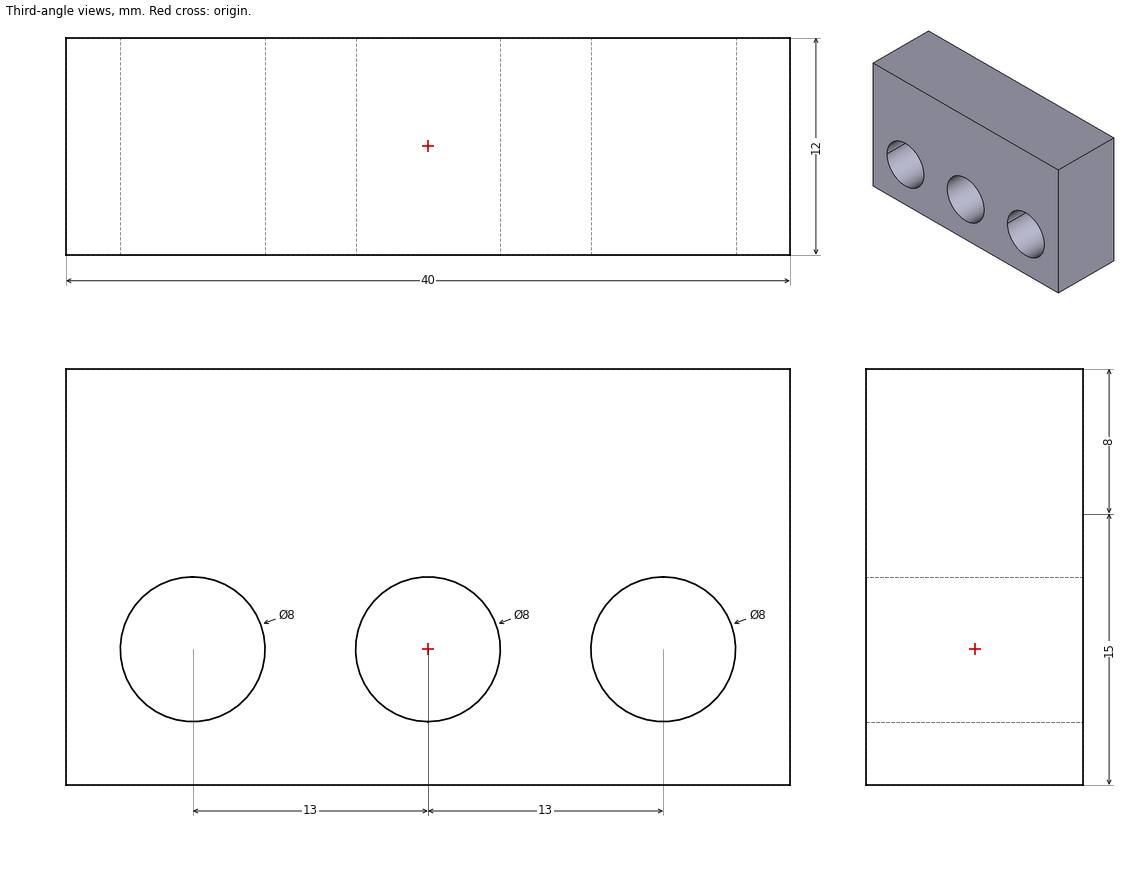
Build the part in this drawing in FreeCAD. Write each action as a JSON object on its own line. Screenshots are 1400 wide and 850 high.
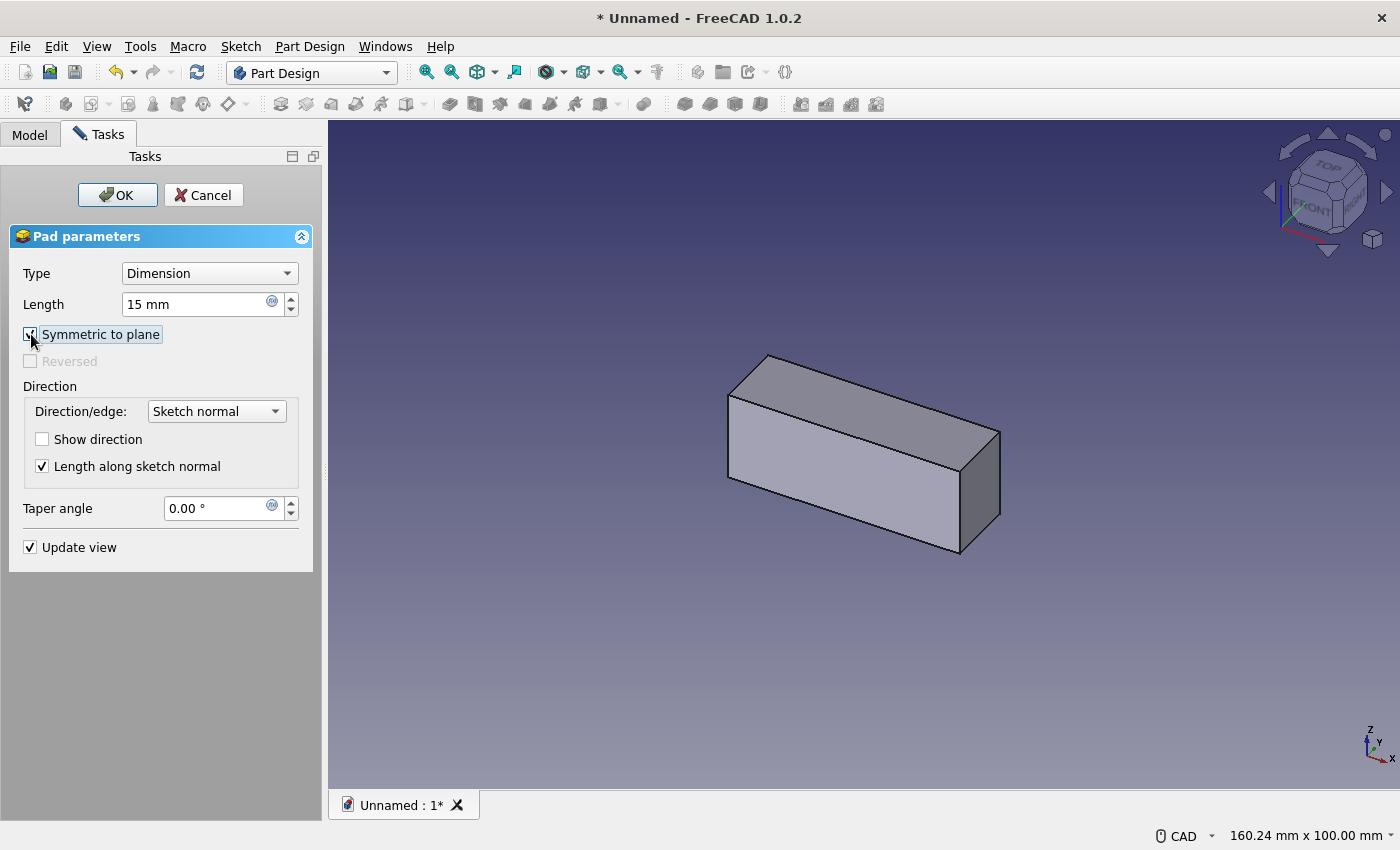
{"action": "left_click", "coordinate": [118, 195]}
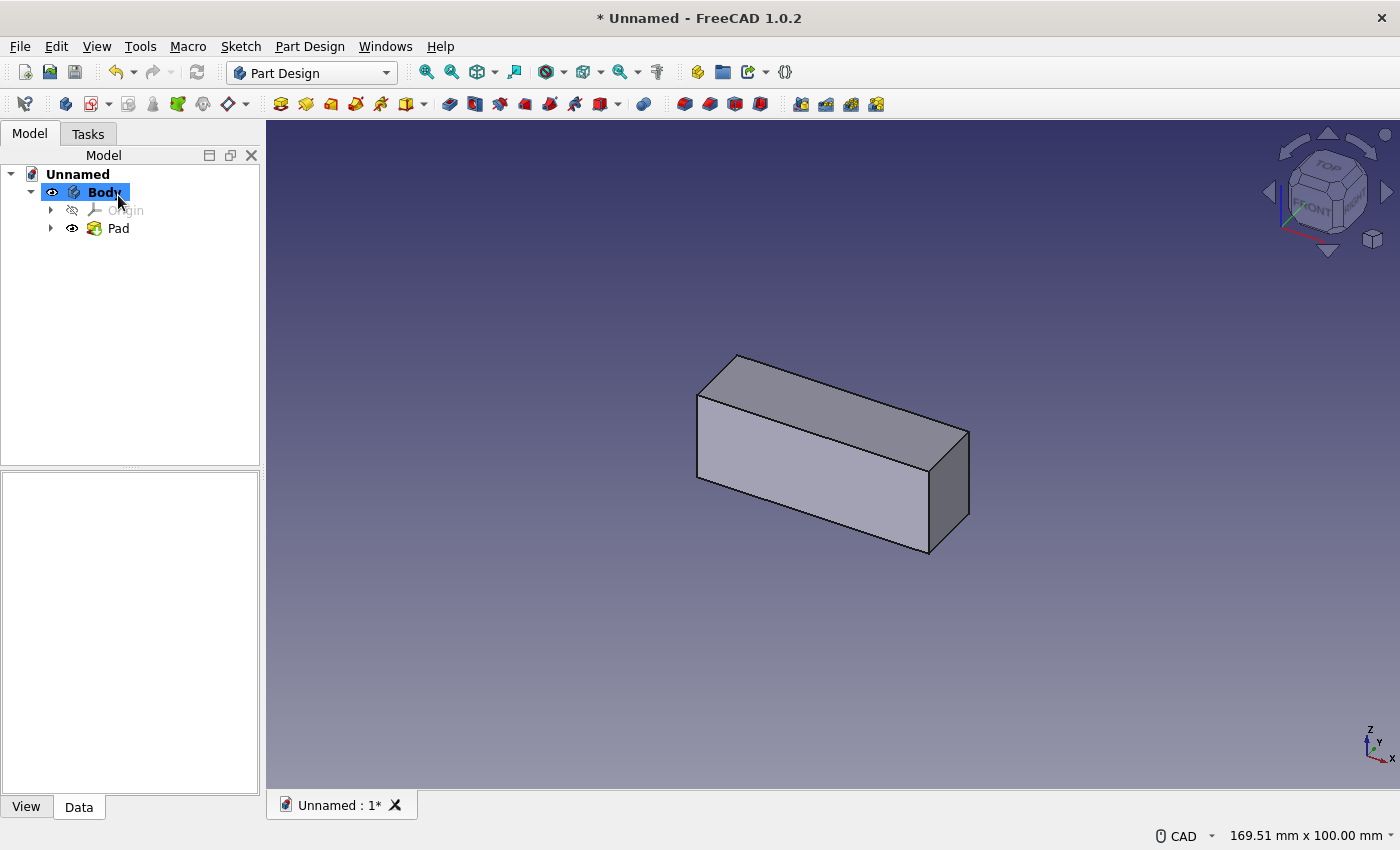
{"action": "key", "text": "v f"}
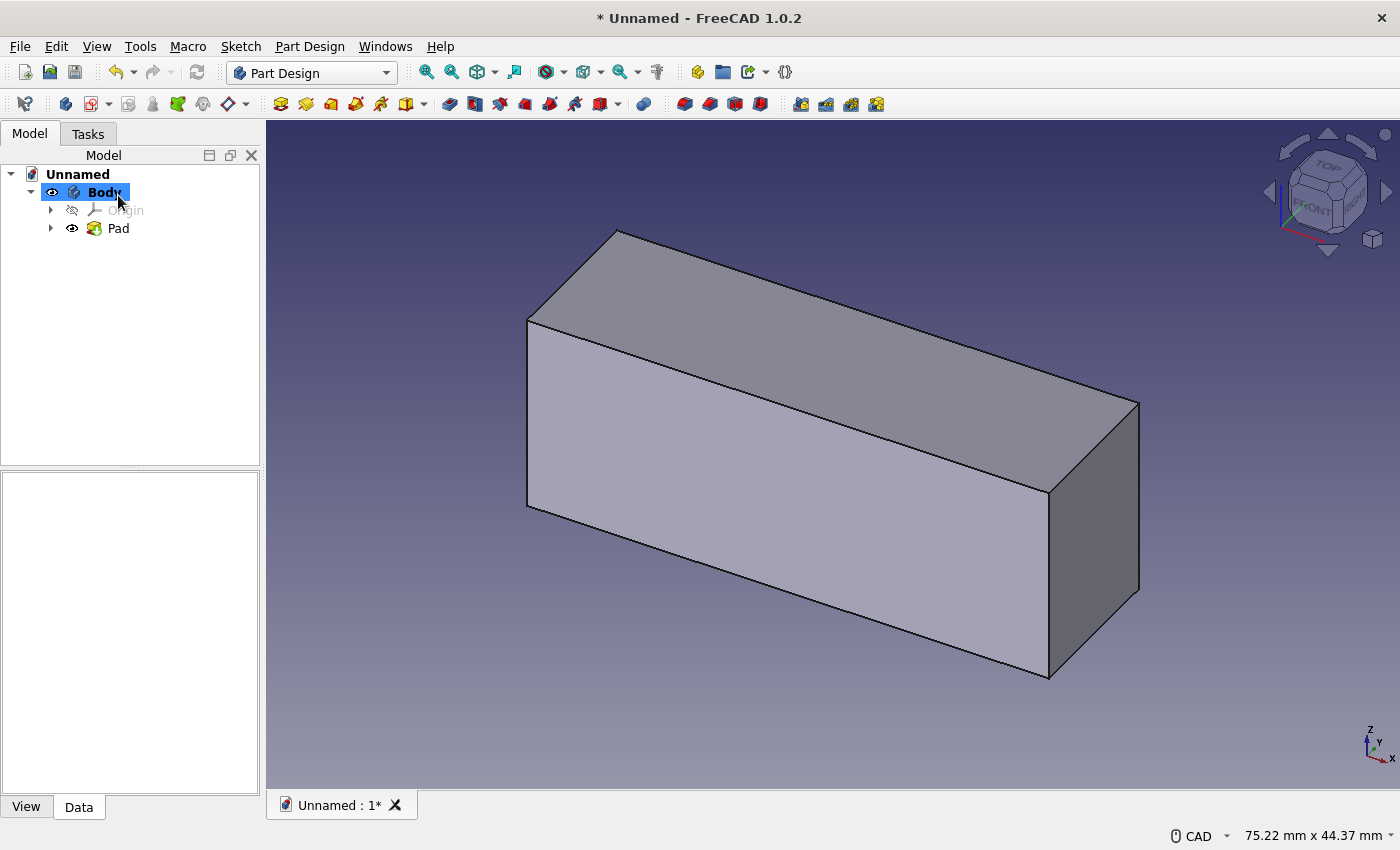
{"action": "key", "text": "4"}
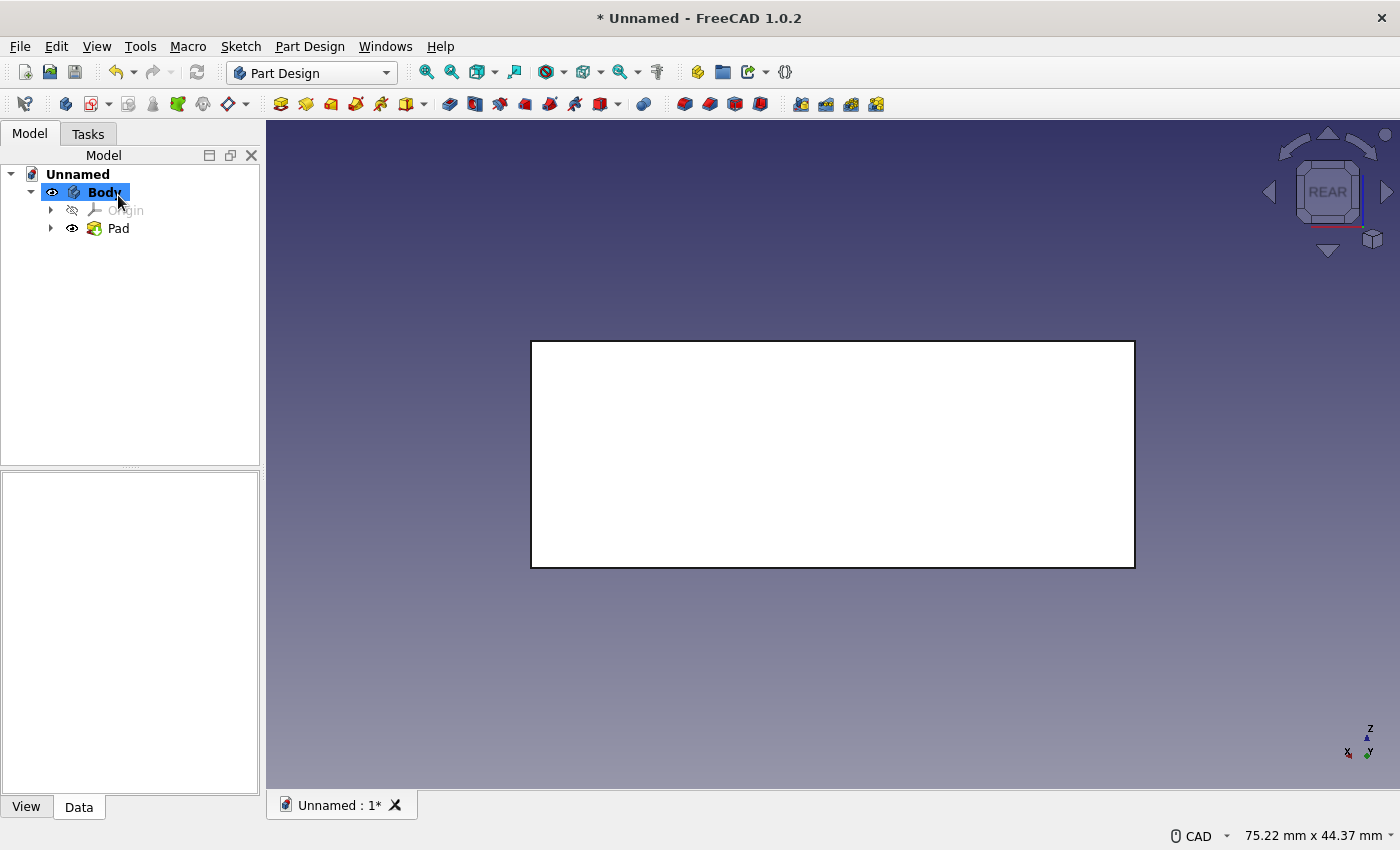
{"action": "left_click", "coordinate": [661, 453]}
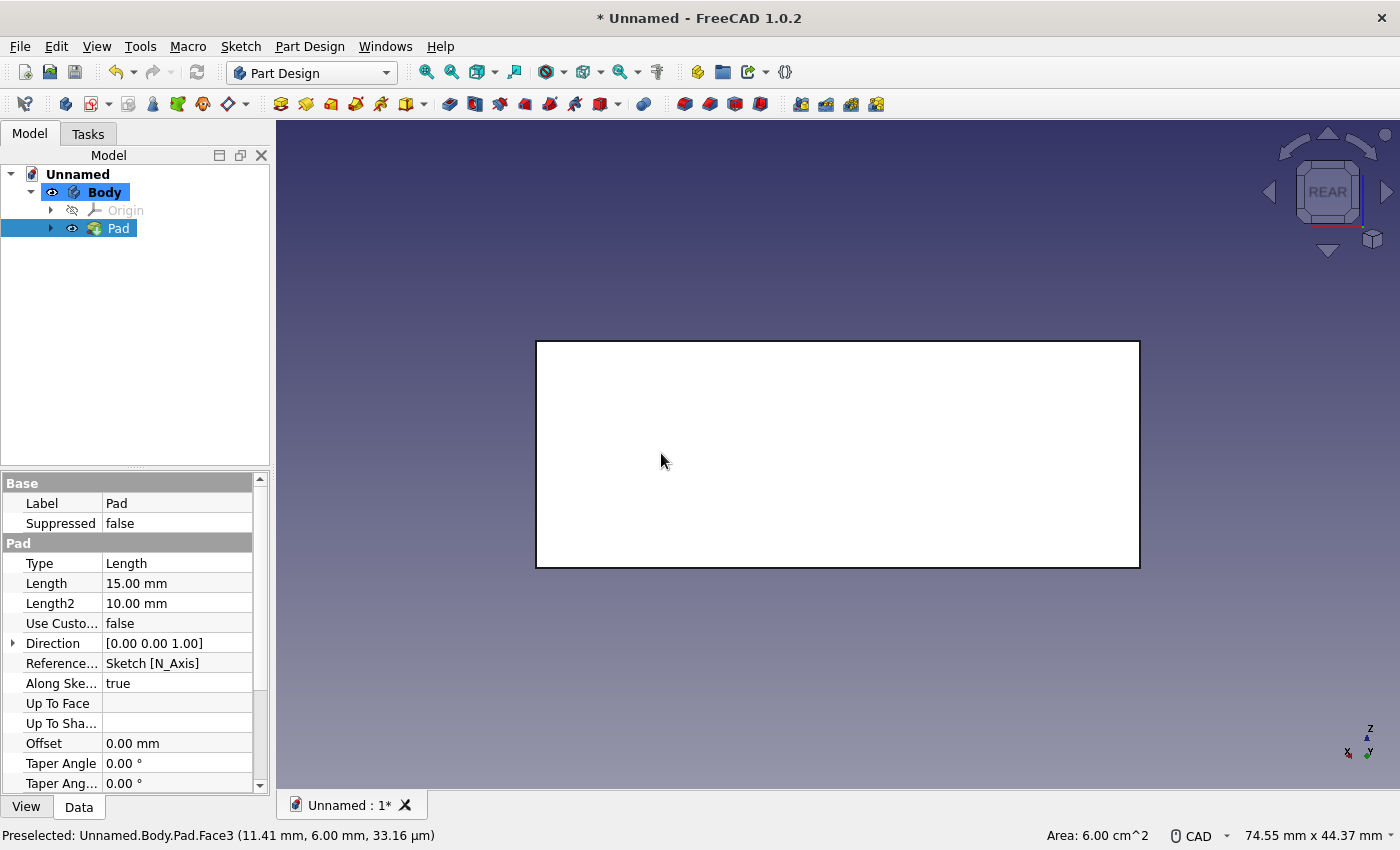
{"action": "left_click", "coordinate": [90, 104]}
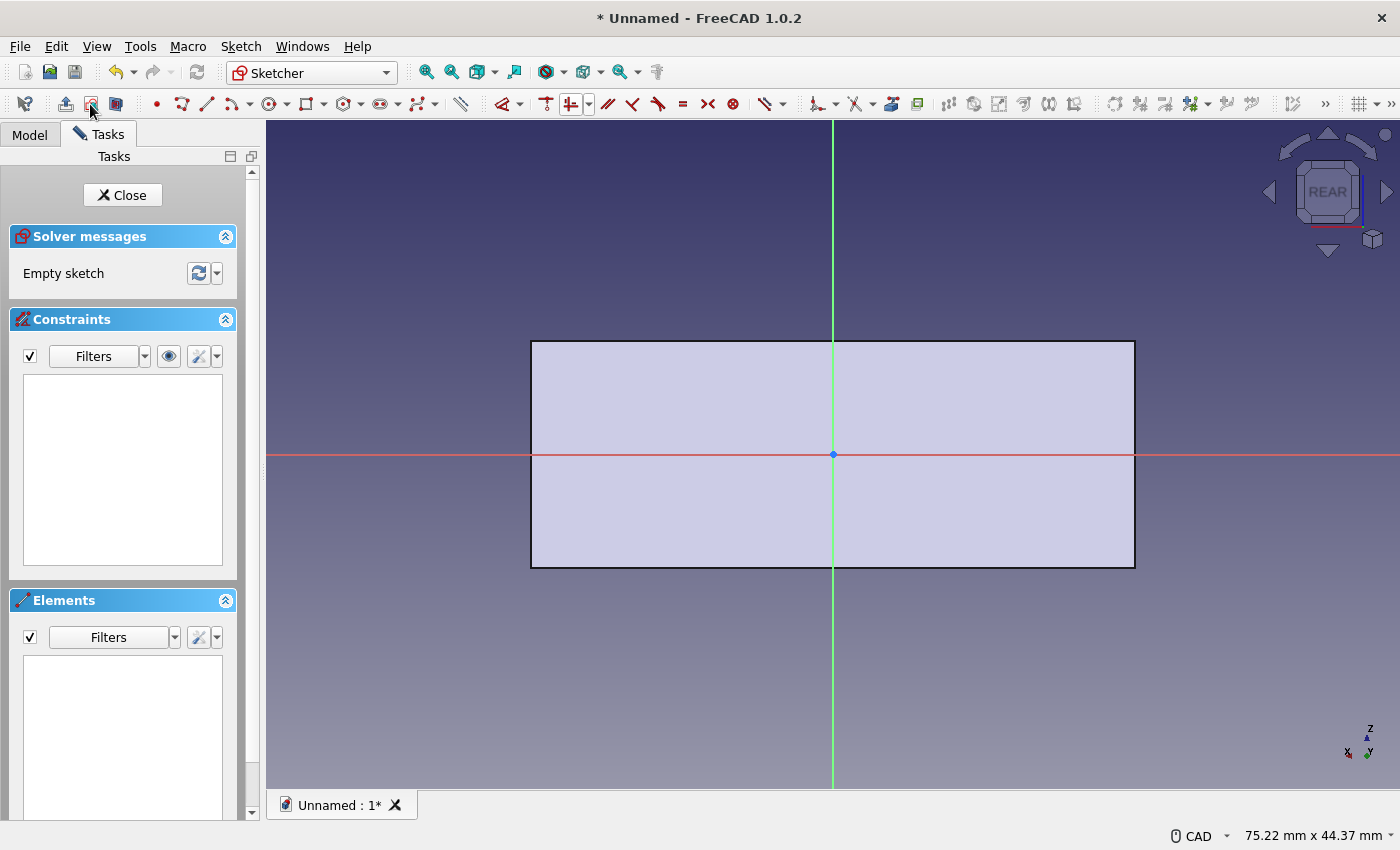
{"action": "scroll", "coordinate": [1076, 454], "scroll_direction": "up", "scroll_amount": 5}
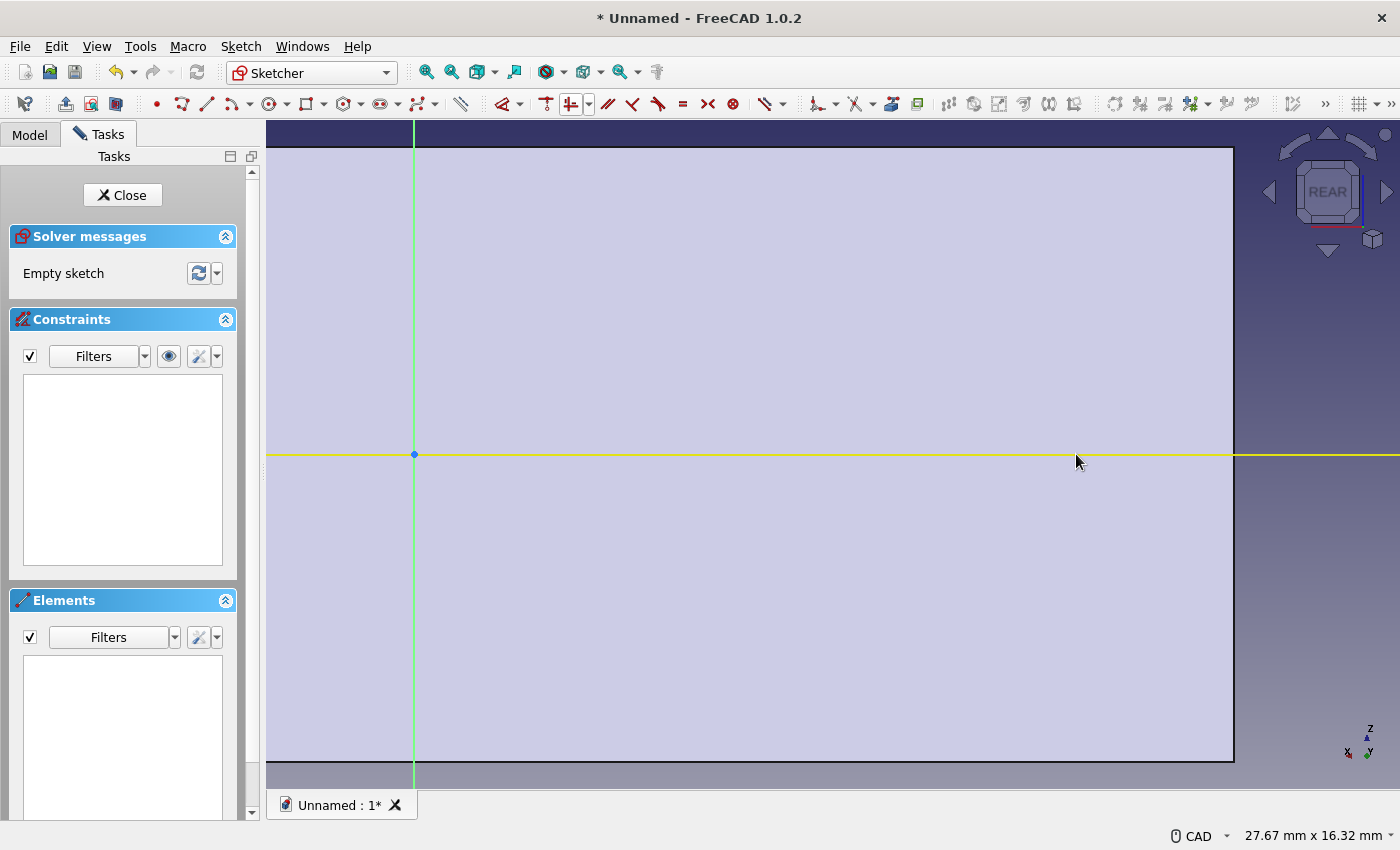
{"action": "key", "text": "g c"}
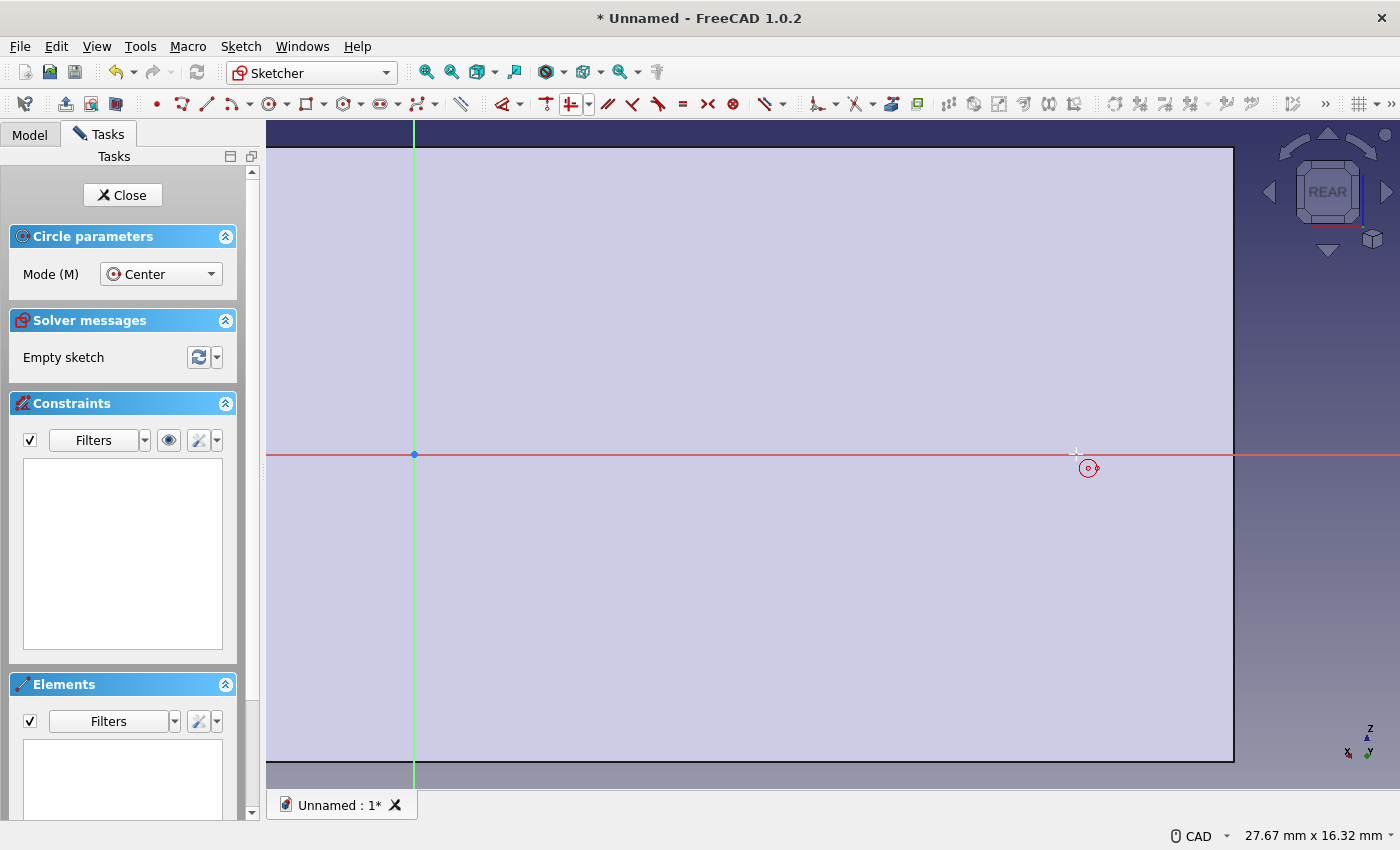
{"action": "left_click", "coordinate": [947, 454]}
{"action": "left_click", "coordinate": [1063, 339]}
{"action": "key", "text": "Escape"}